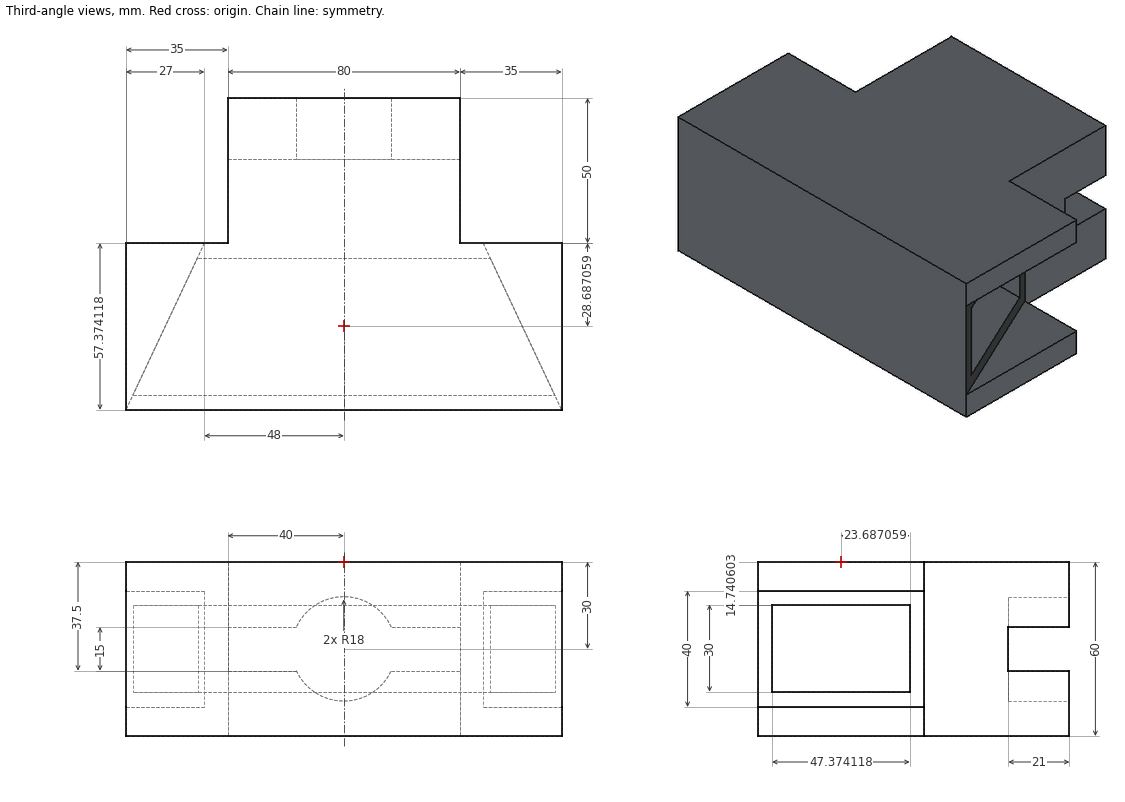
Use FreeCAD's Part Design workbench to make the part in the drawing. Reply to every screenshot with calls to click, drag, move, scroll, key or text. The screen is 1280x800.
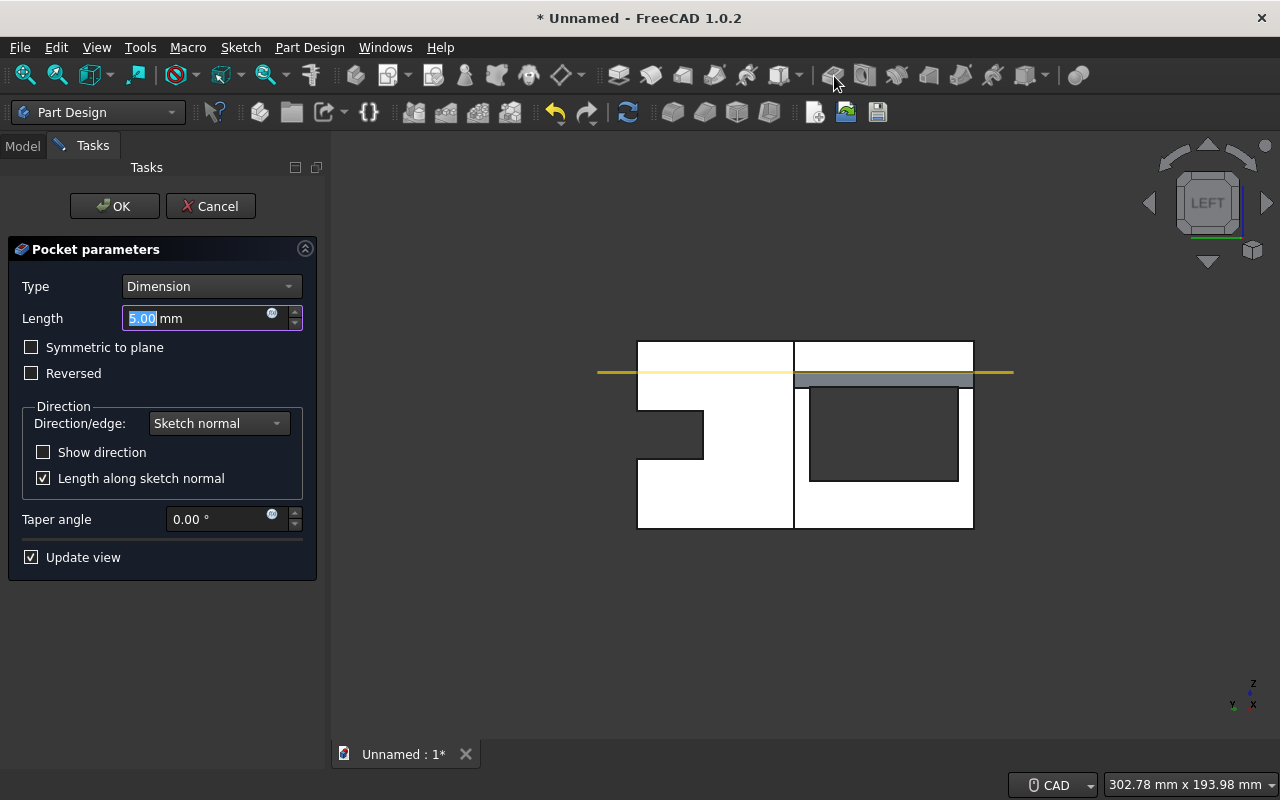
text(40)
key(Tab)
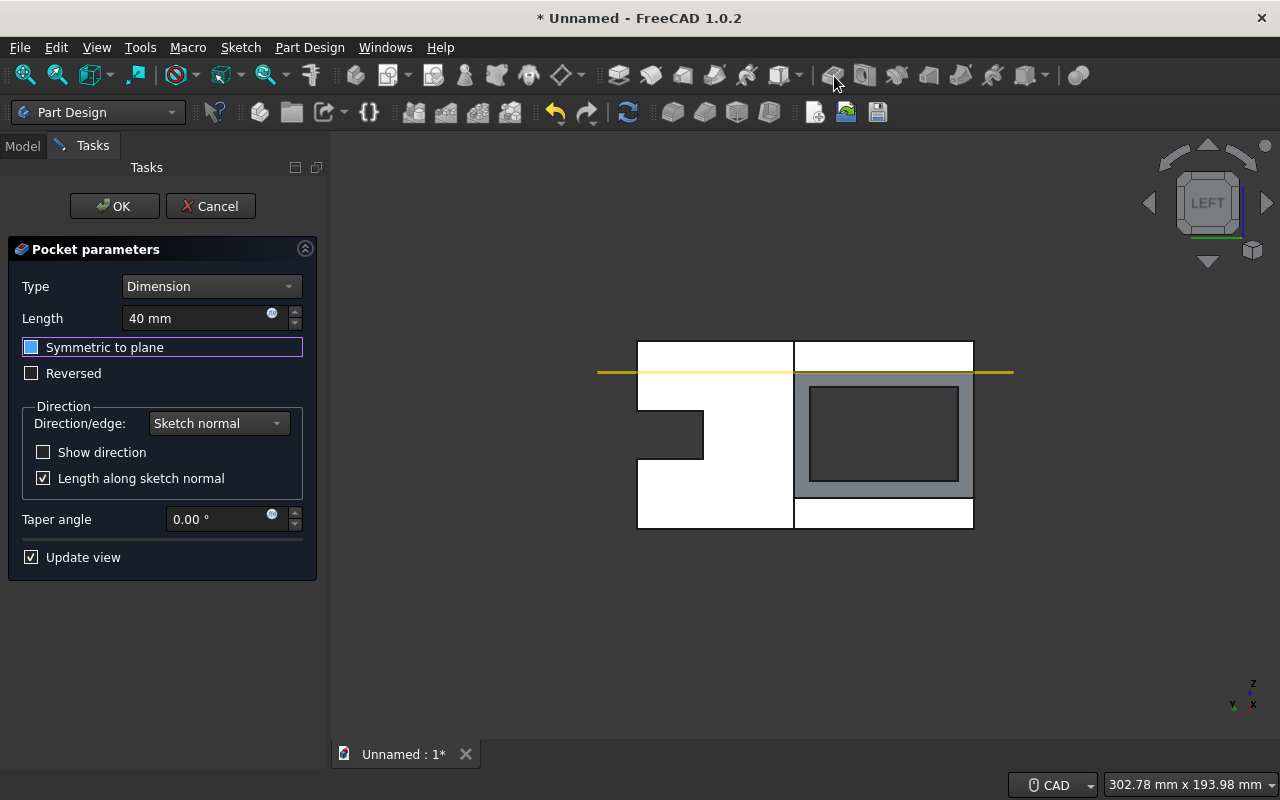
click(115, 206)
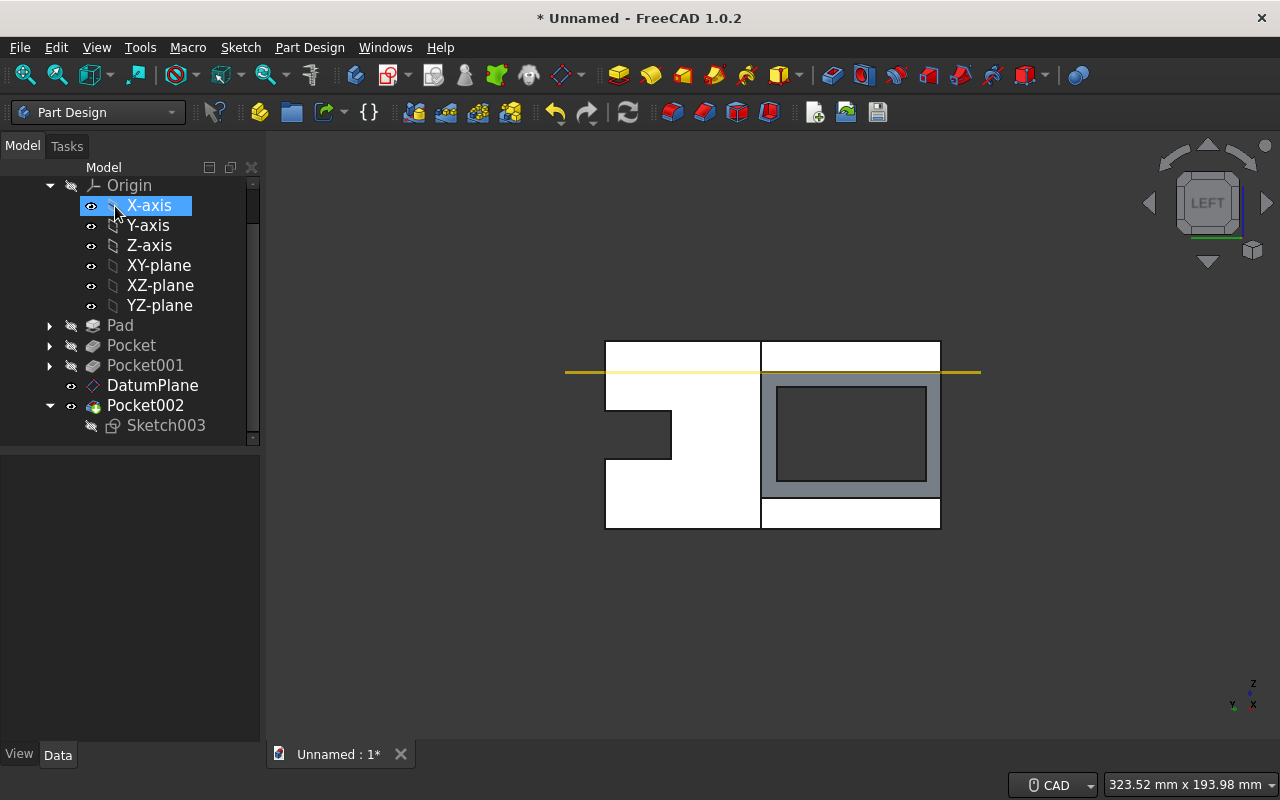
click(116, 386)
key(space)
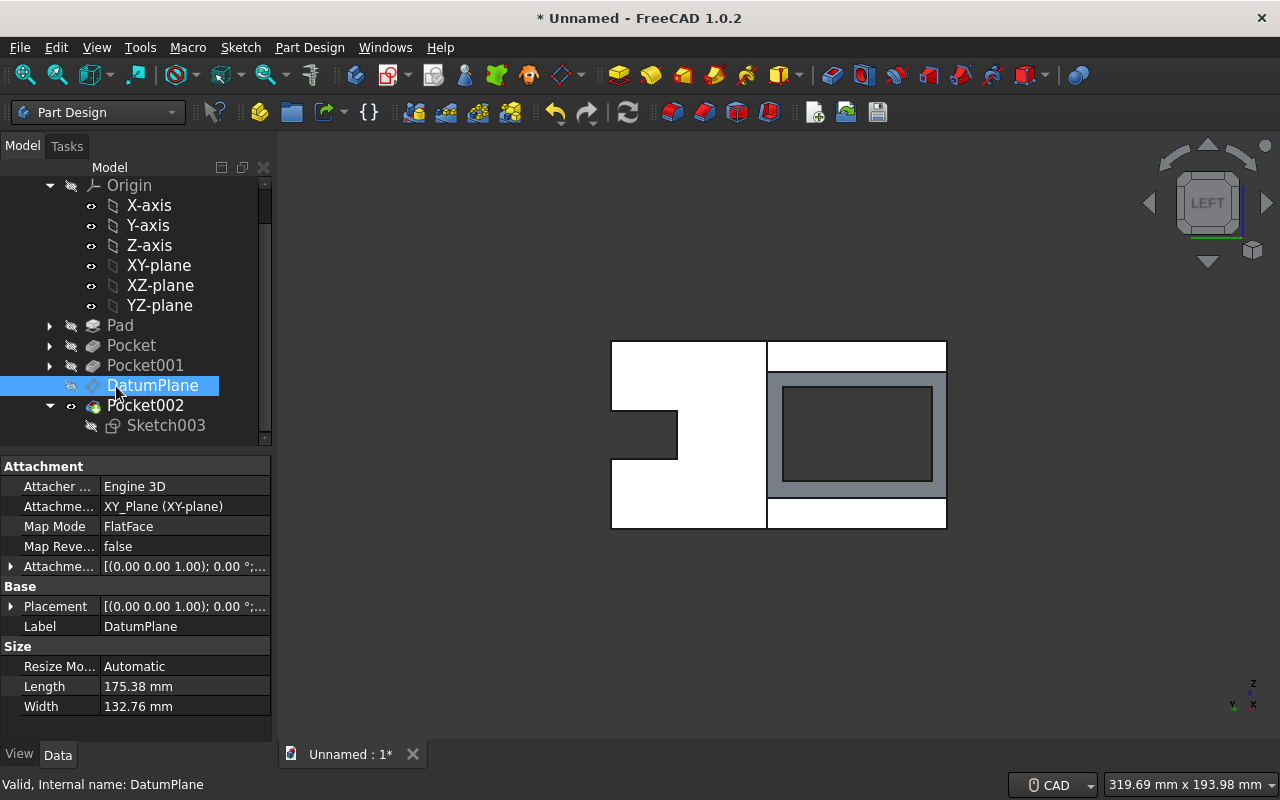
key(0)